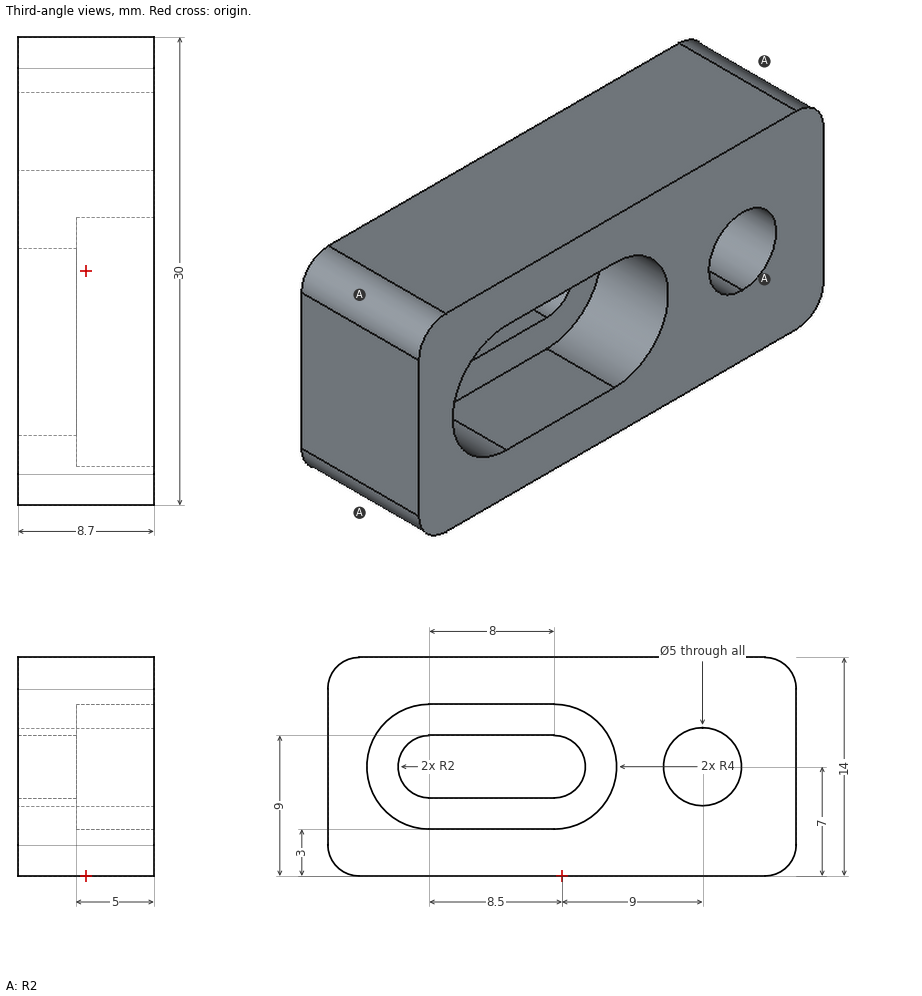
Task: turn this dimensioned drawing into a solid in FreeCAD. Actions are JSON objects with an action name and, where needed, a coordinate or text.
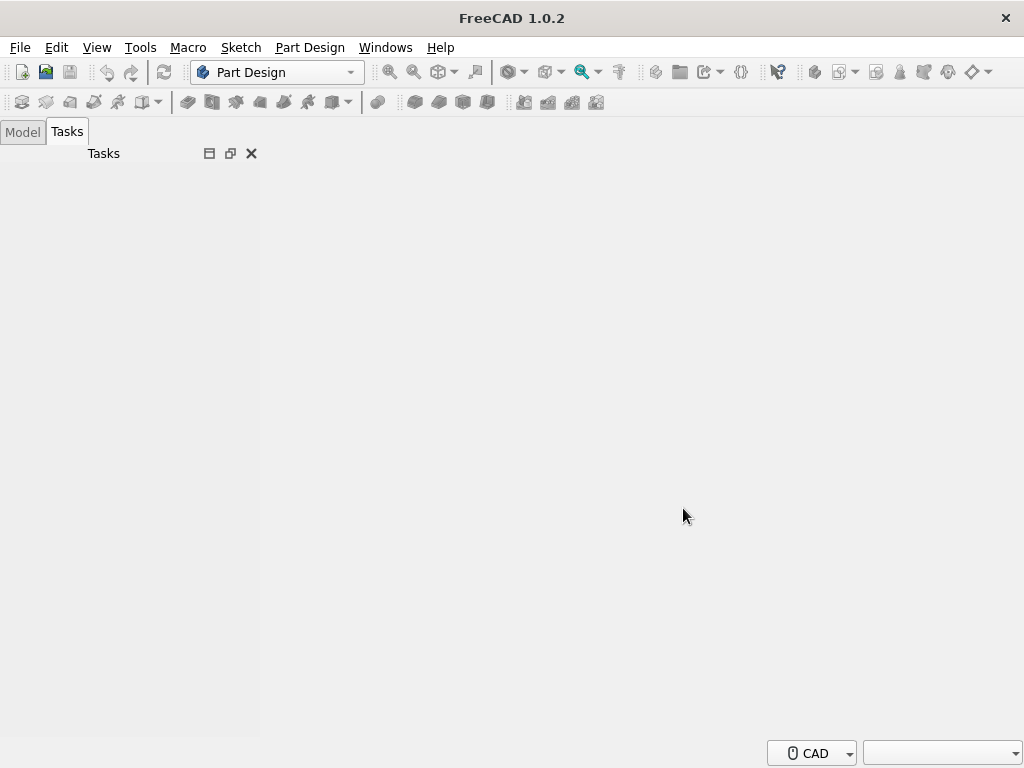
{"action": "left_click", "coordinate": [22, 72]}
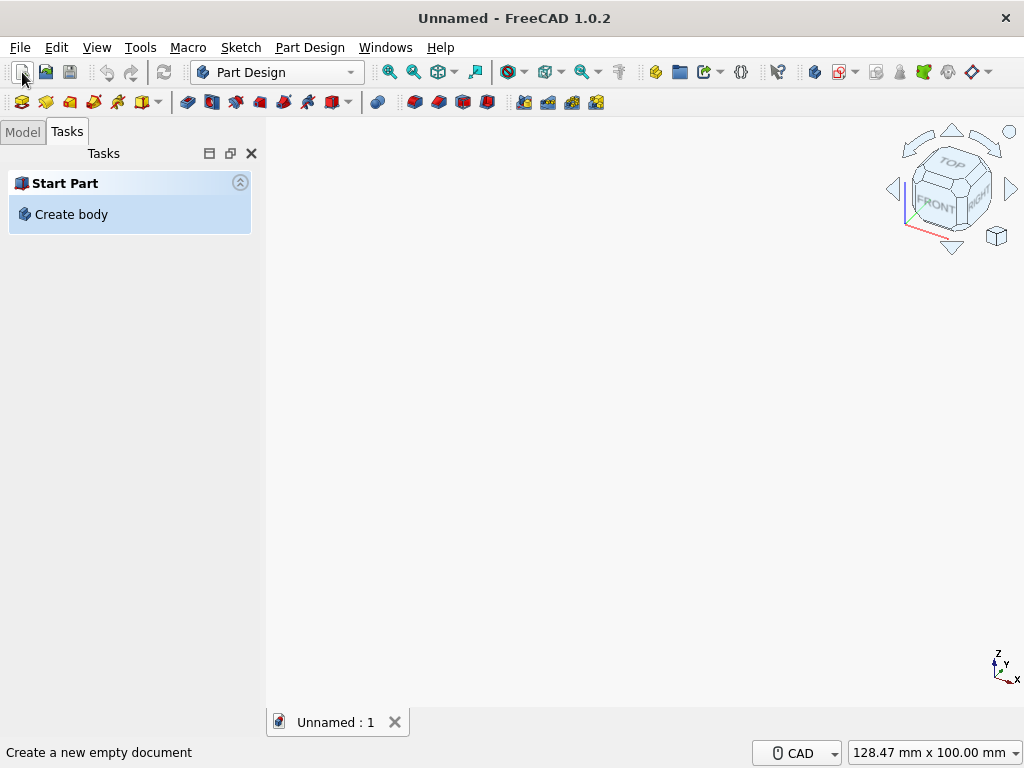
{"action": "left_click", "coordinate": [840, 72]}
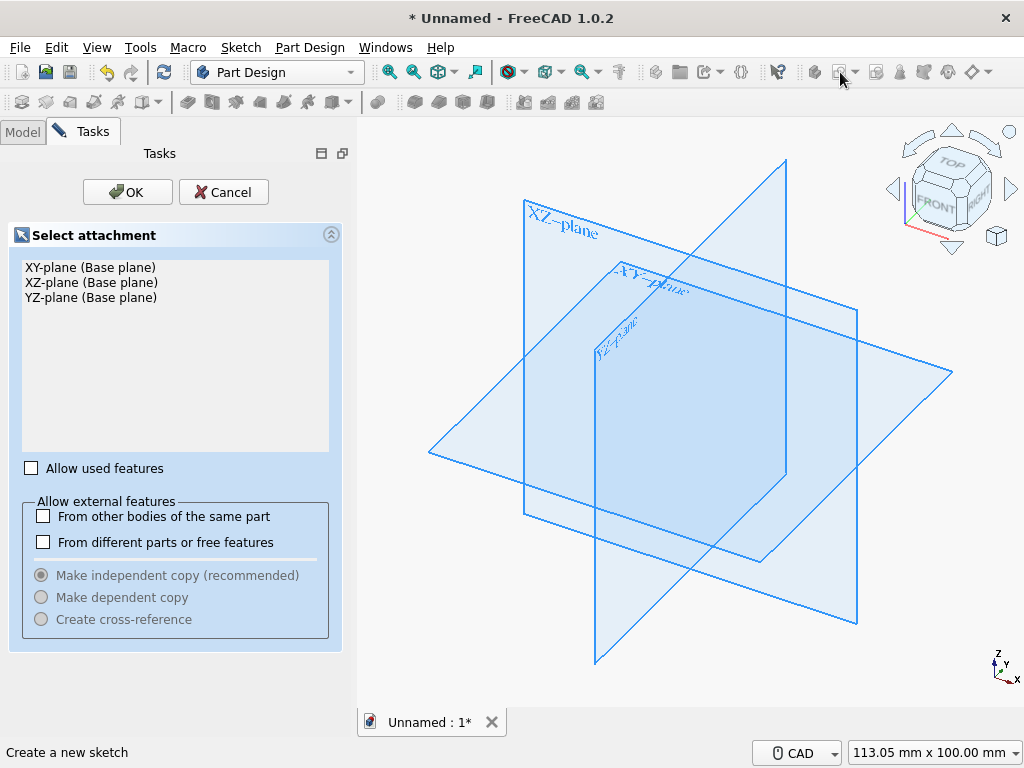
{"action": "left_click", "coordinate": [82, 268]}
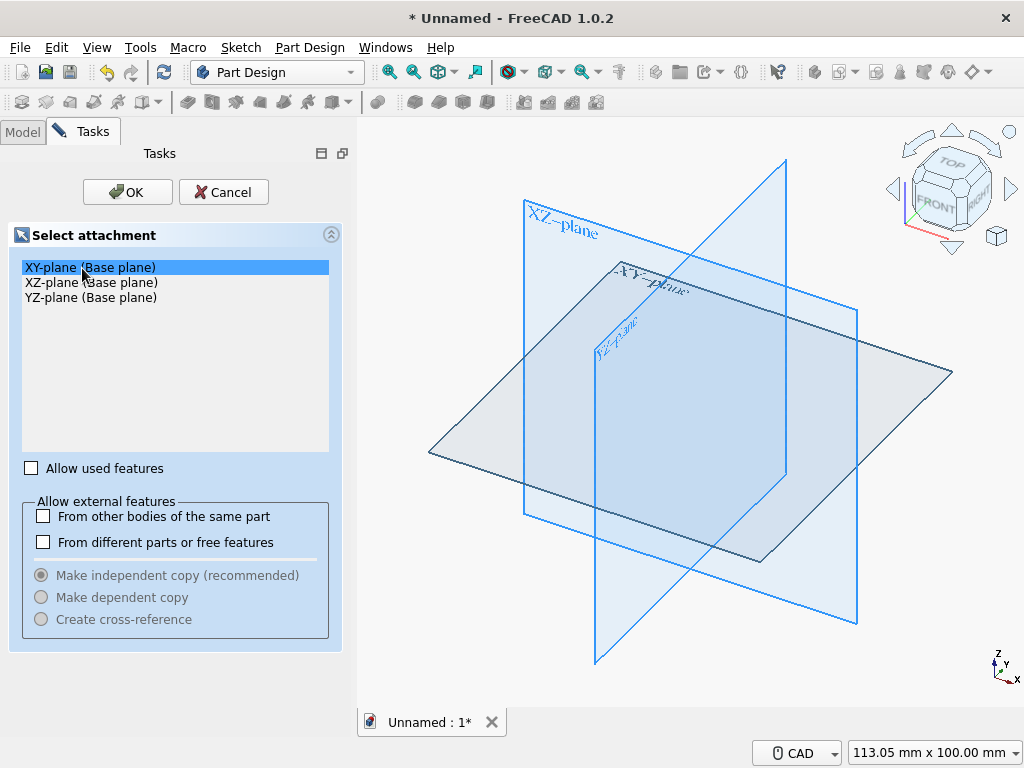
{"action": "left_click", "coordinate": [128, 192]}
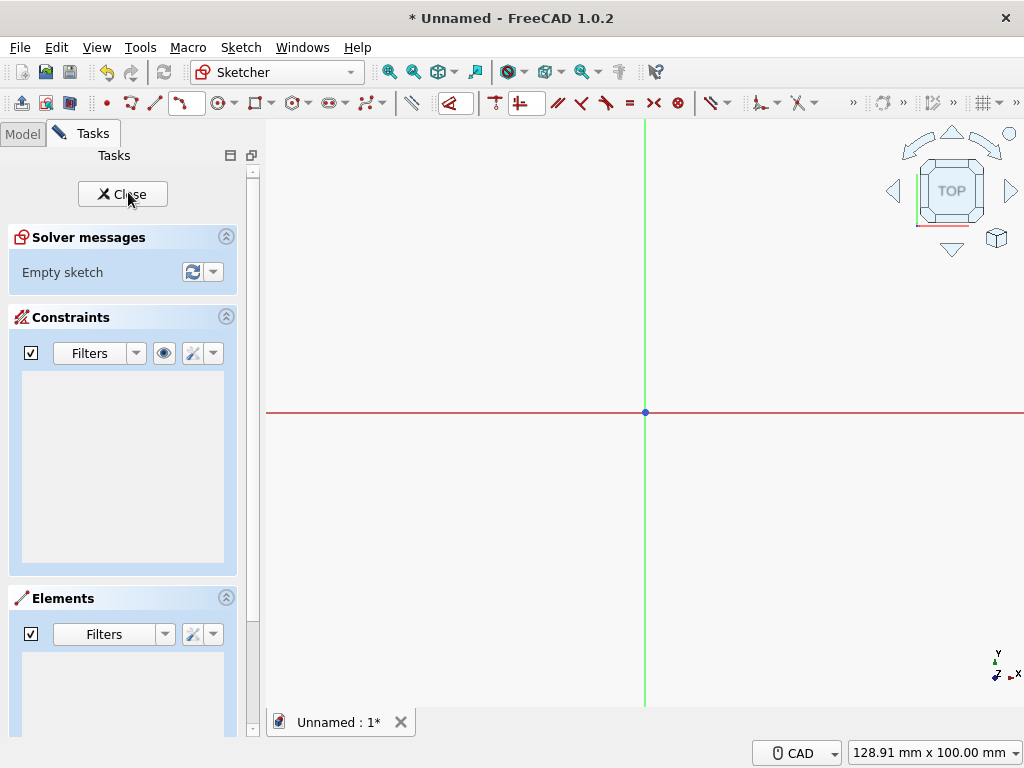
{"action": "scroll", "coordinate": [701, 413], "scroll_direction": "up", "scroll_amount": 4}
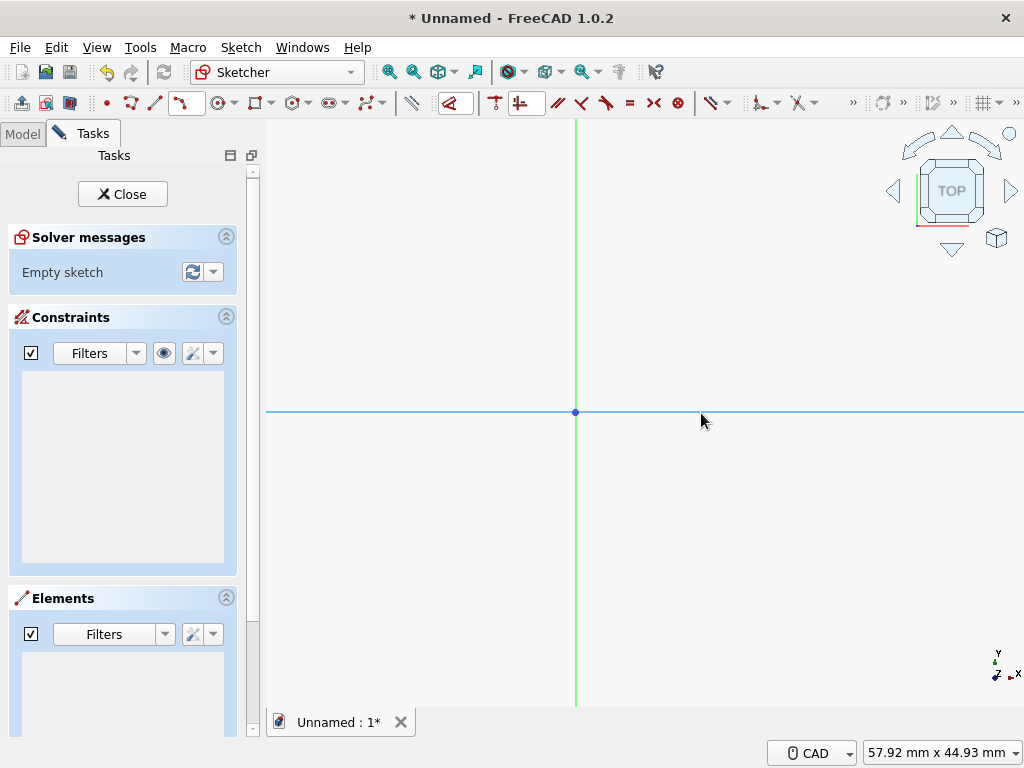
{"action": "left_click", "coordinate": [274, 104]}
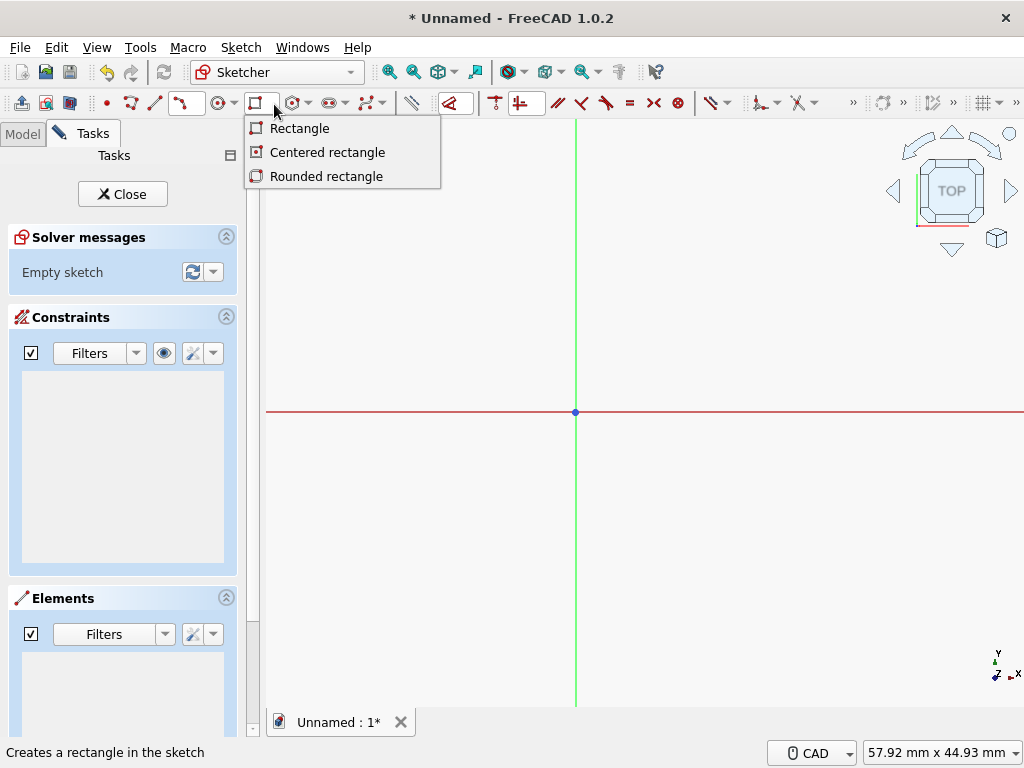
{"action": "left_click", "coordinate": [342, 152]}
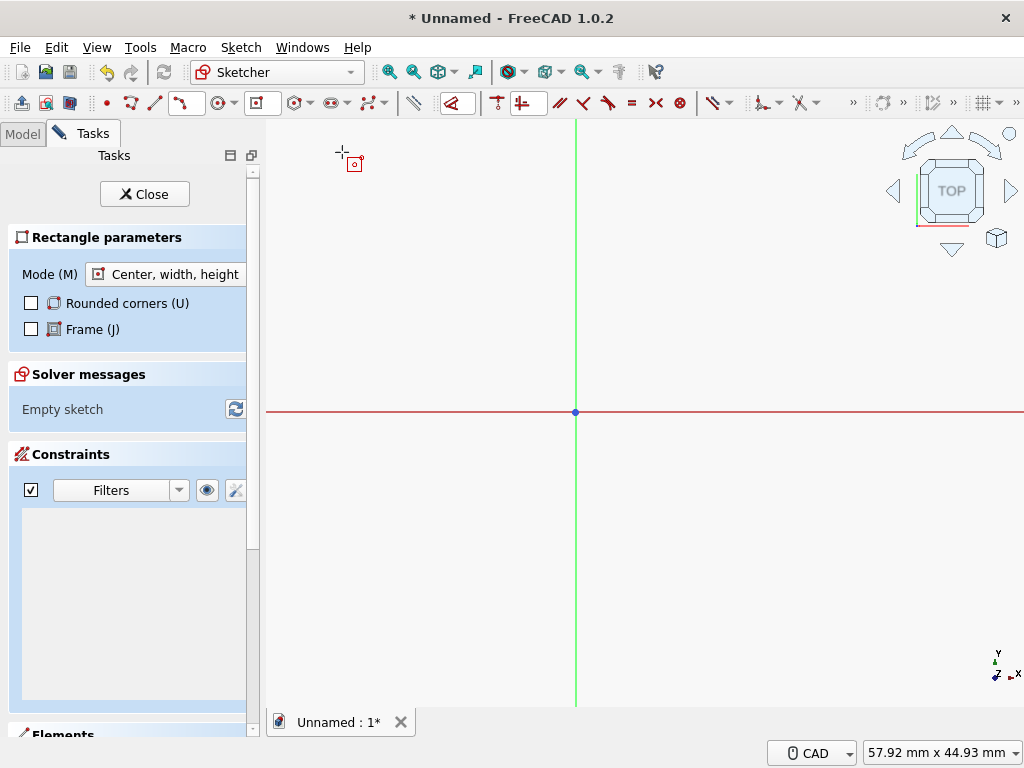
{"action": "left_click", "coordinate": [576, 412]}
{"action": "left_click", "coordinate": [633, 216]}
{"action": "key", "text": "Escape"}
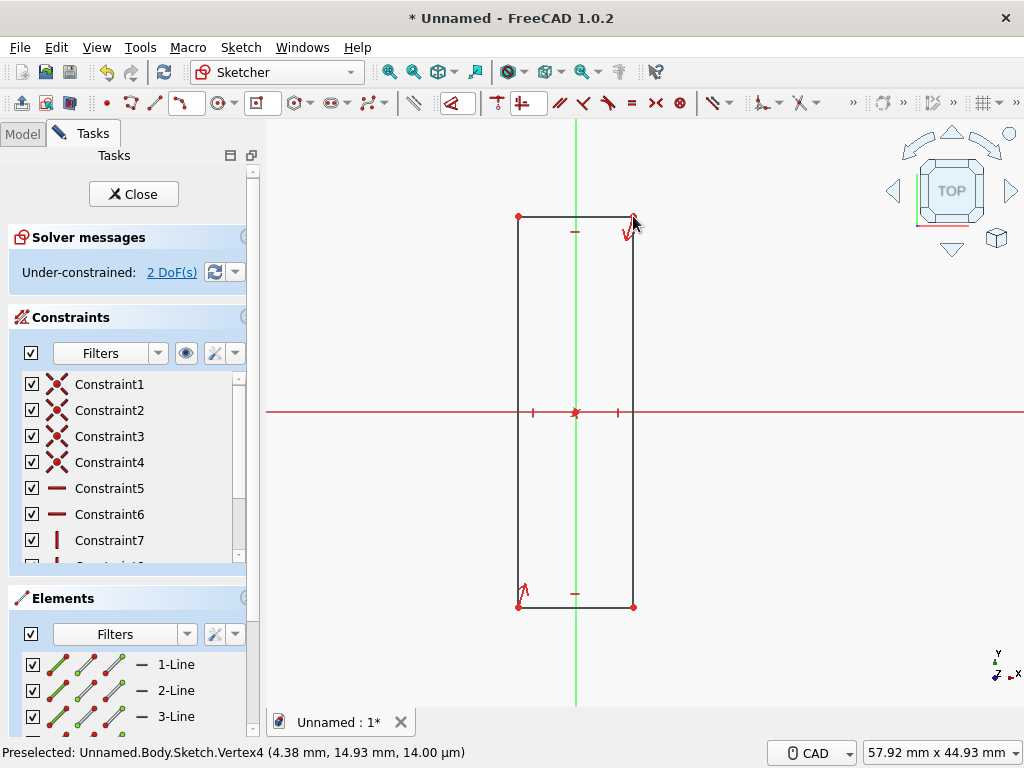
{"action": "left_click", "coordinate": [452, 104]}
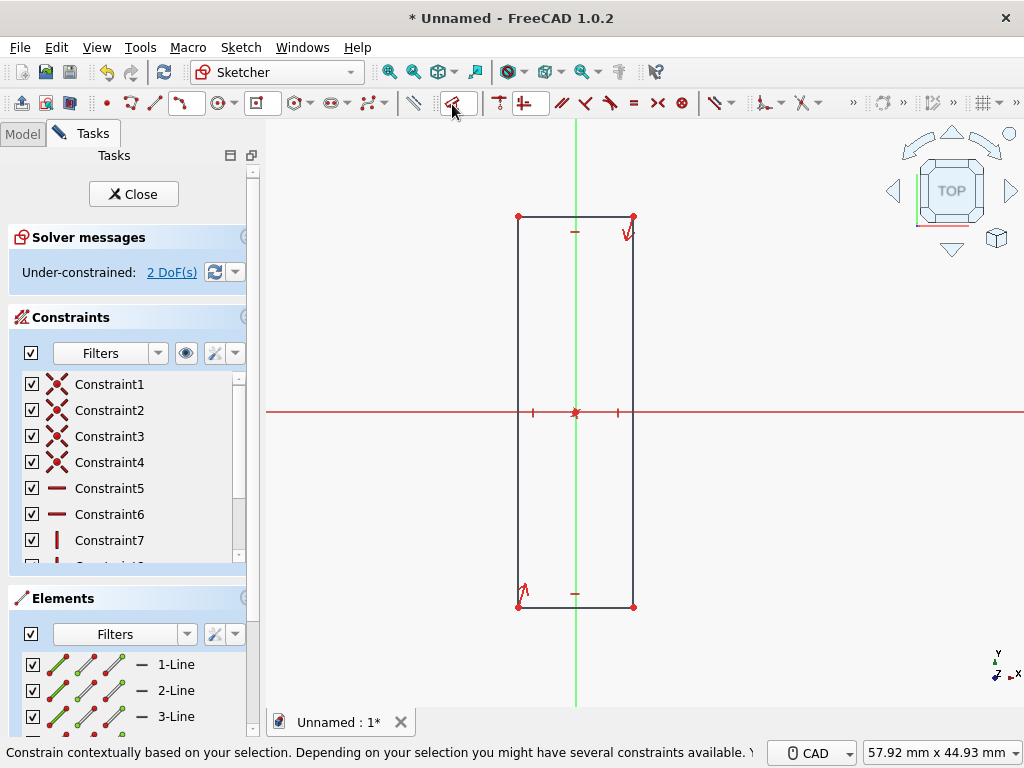
{"action": "left_click", "coordinate": [633, 491]}
{"action": "left_click", "coordinate": [667, 323]}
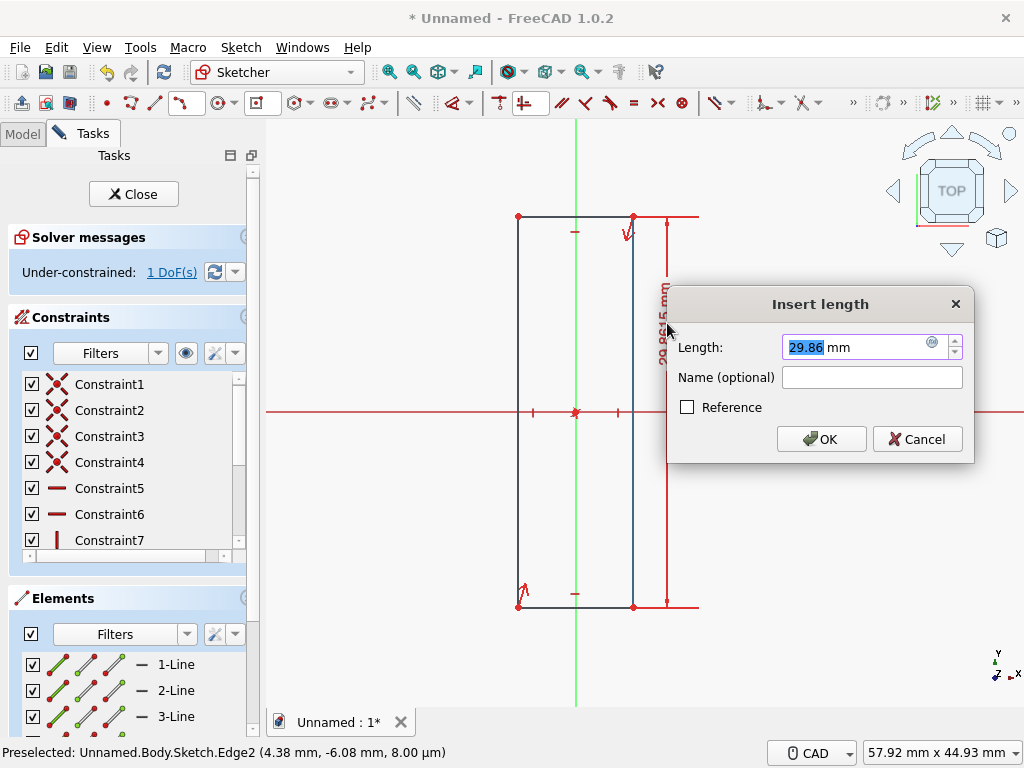
{"action": "type", "text": "30"}
{"action": "key", "text": "Return"}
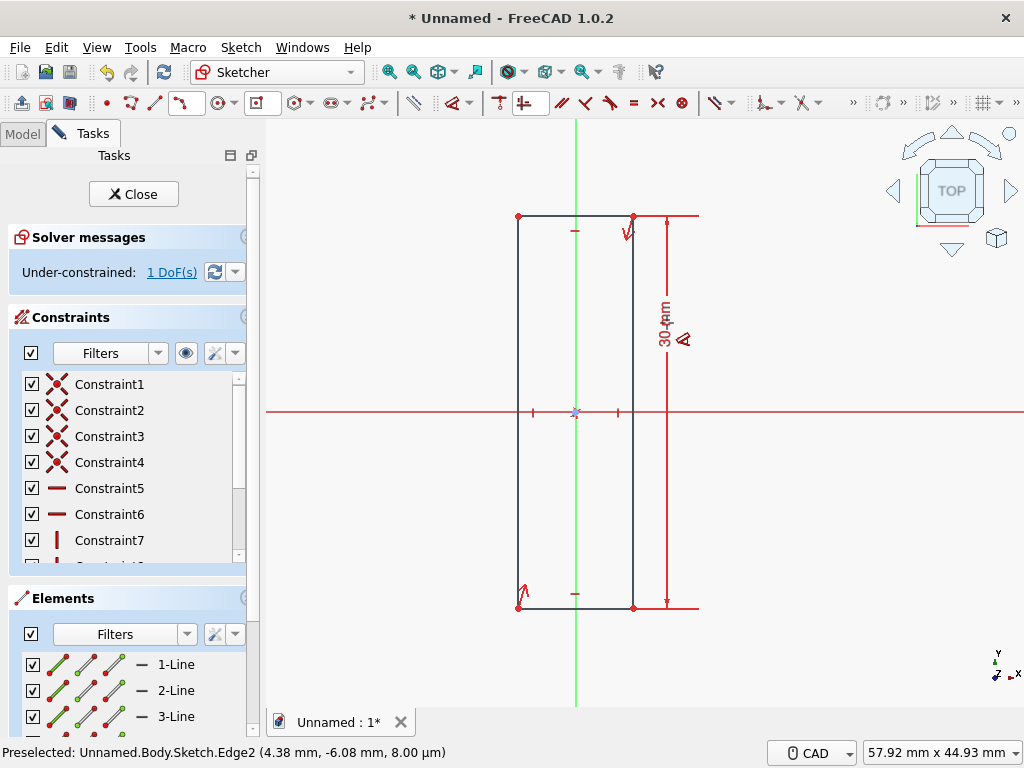
{"action": "left_click", "coordinate": [553, 609]}
{"action": "left_click", "coordinate": [549, 643]}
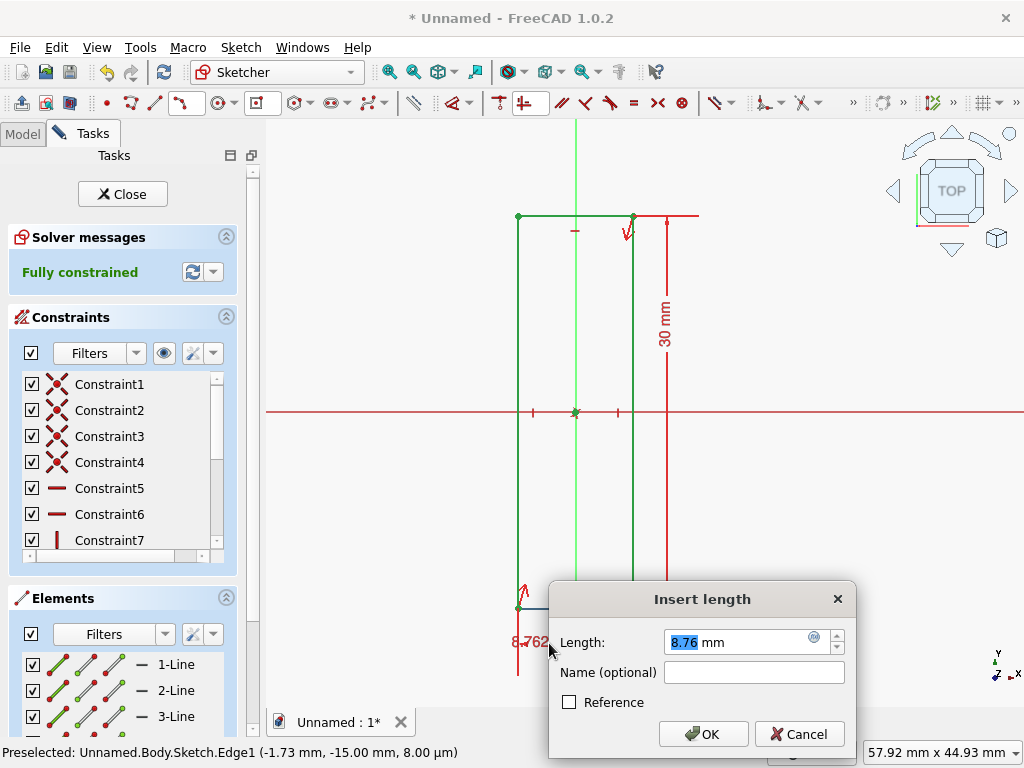
{"action": "type", "text": "8.7"}
{"action": "key", "text": "Return"}
{"action": "key", "text": "Escape"}